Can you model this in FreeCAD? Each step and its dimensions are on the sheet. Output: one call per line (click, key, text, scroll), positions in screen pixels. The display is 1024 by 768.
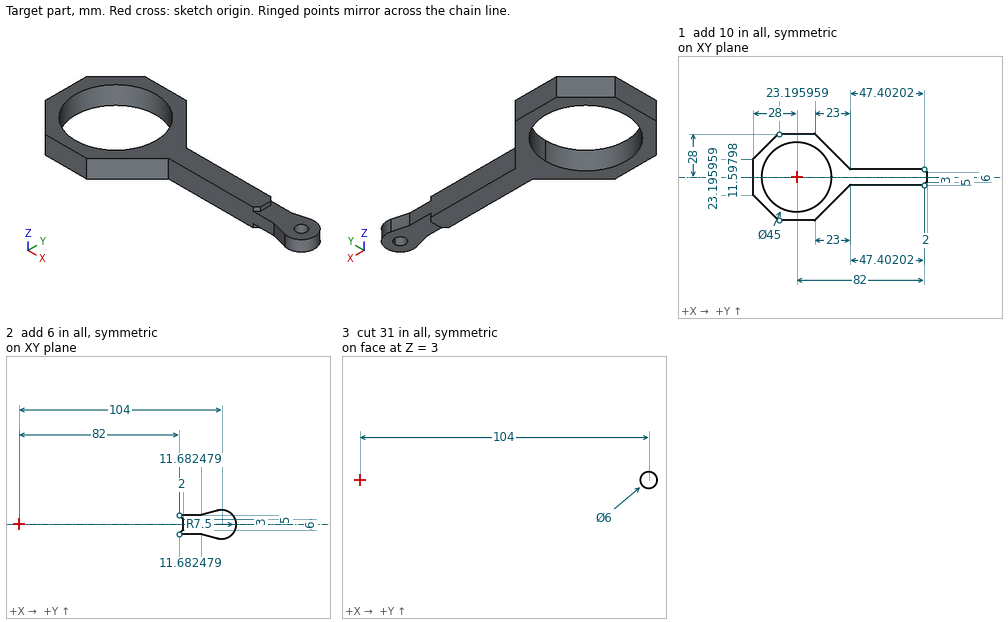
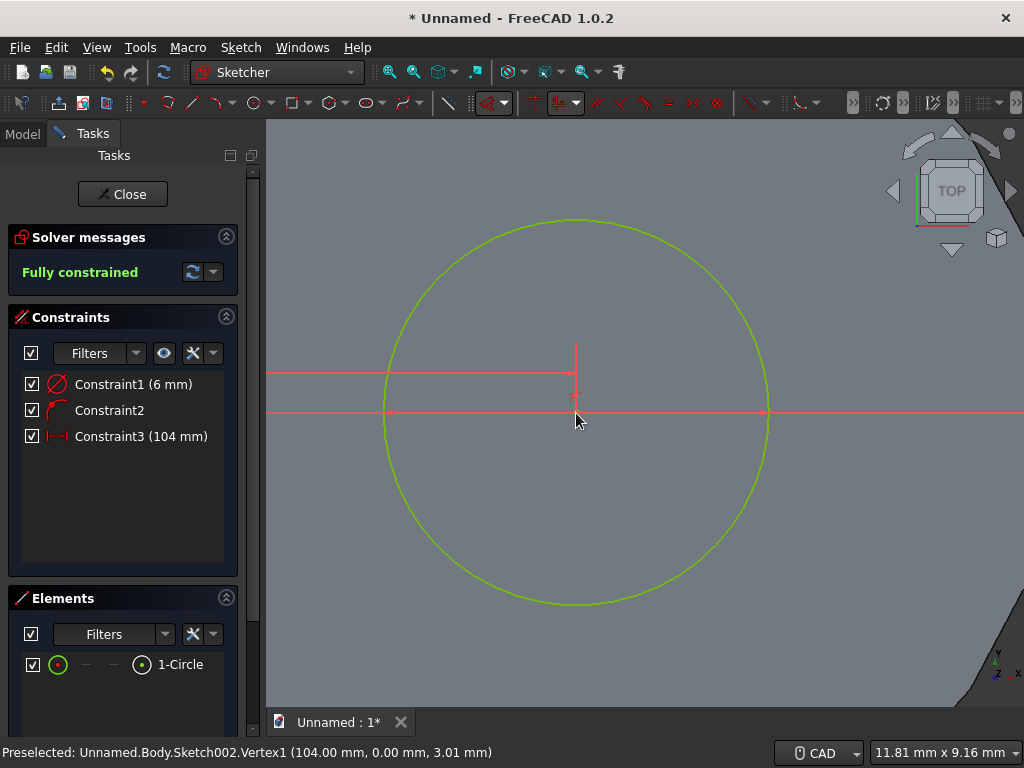
click(123, 194)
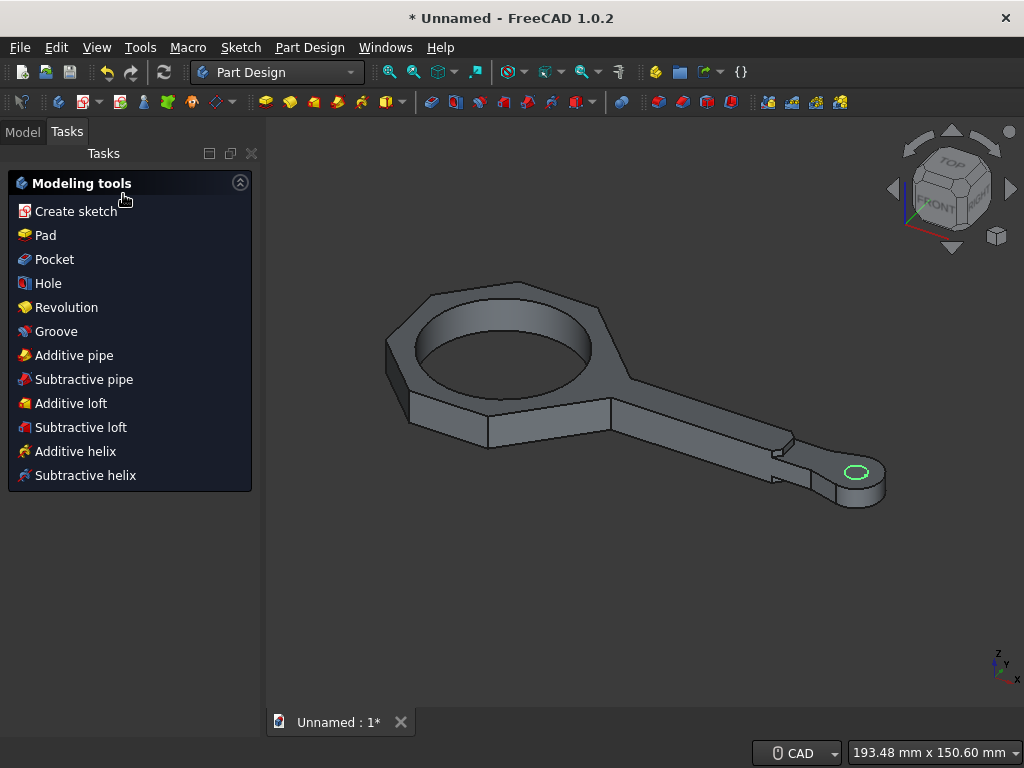
click(432, 102)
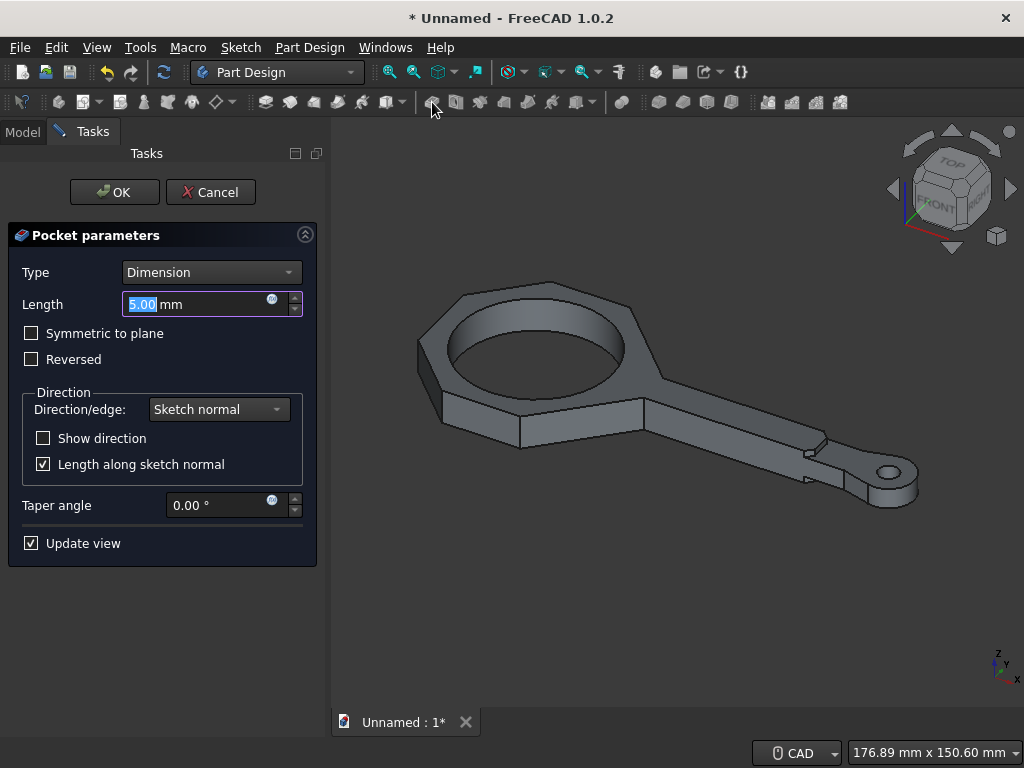
text(31)
key(Tab)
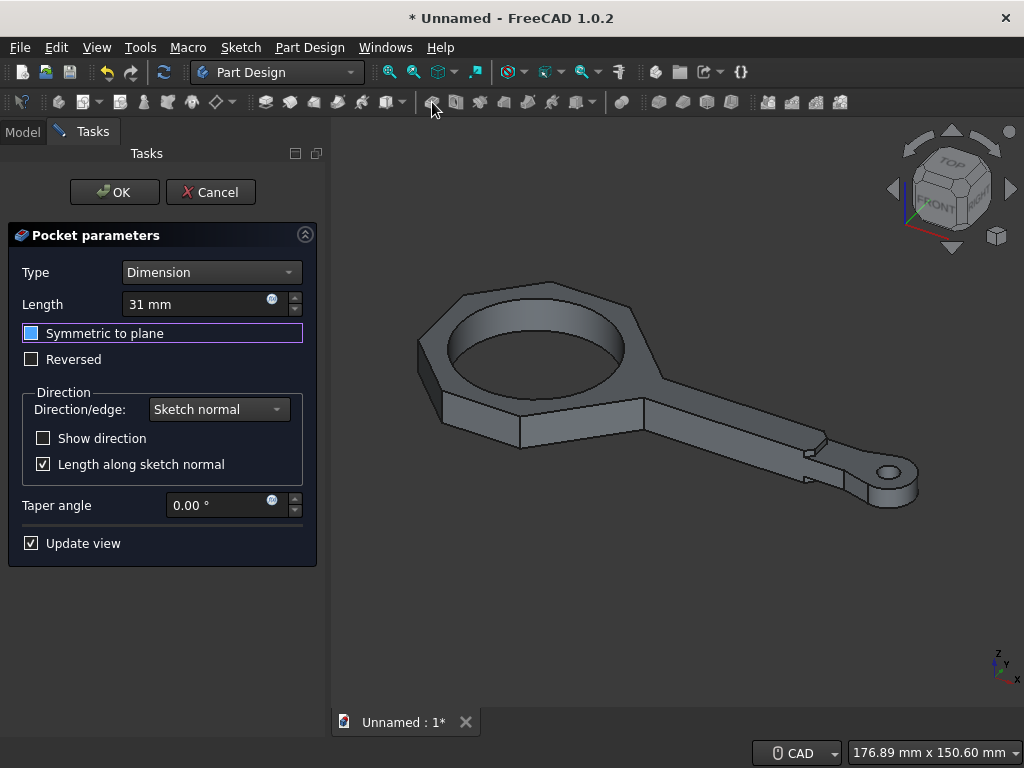
click(30, 333)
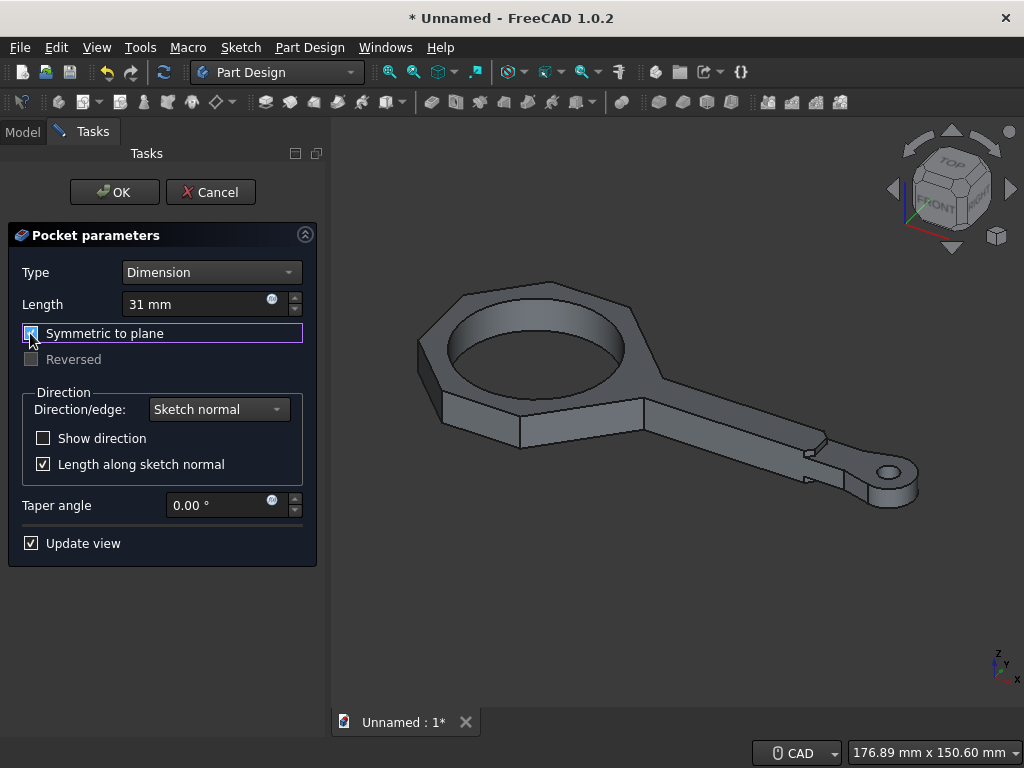
click(115, 192)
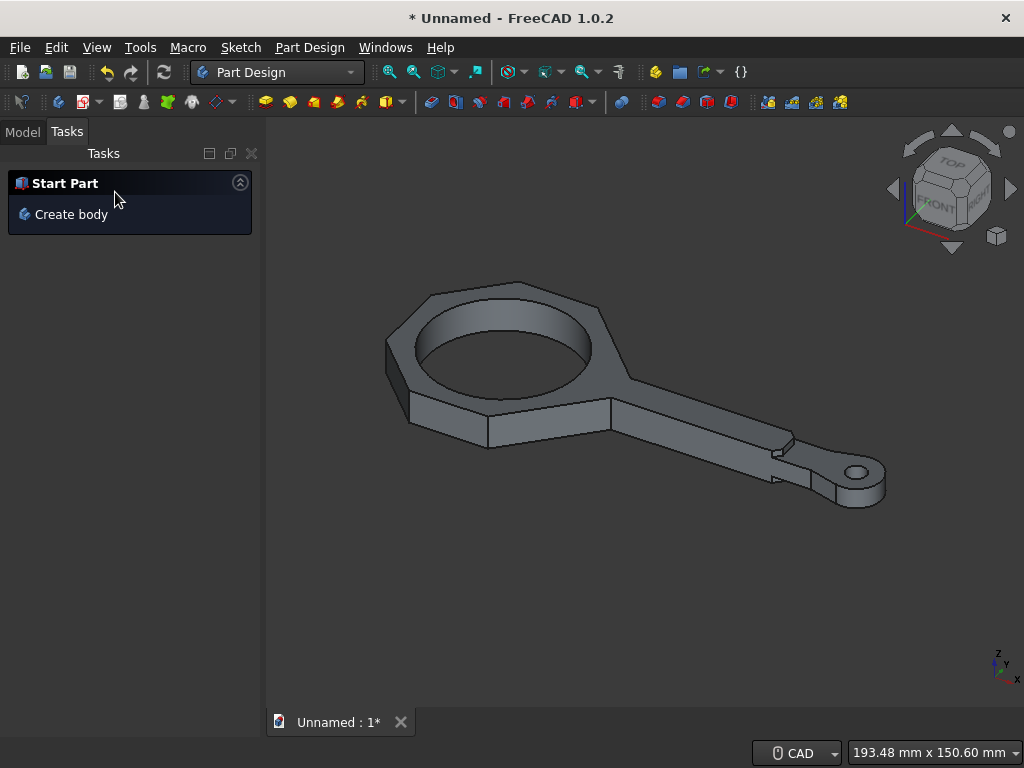
key(0)